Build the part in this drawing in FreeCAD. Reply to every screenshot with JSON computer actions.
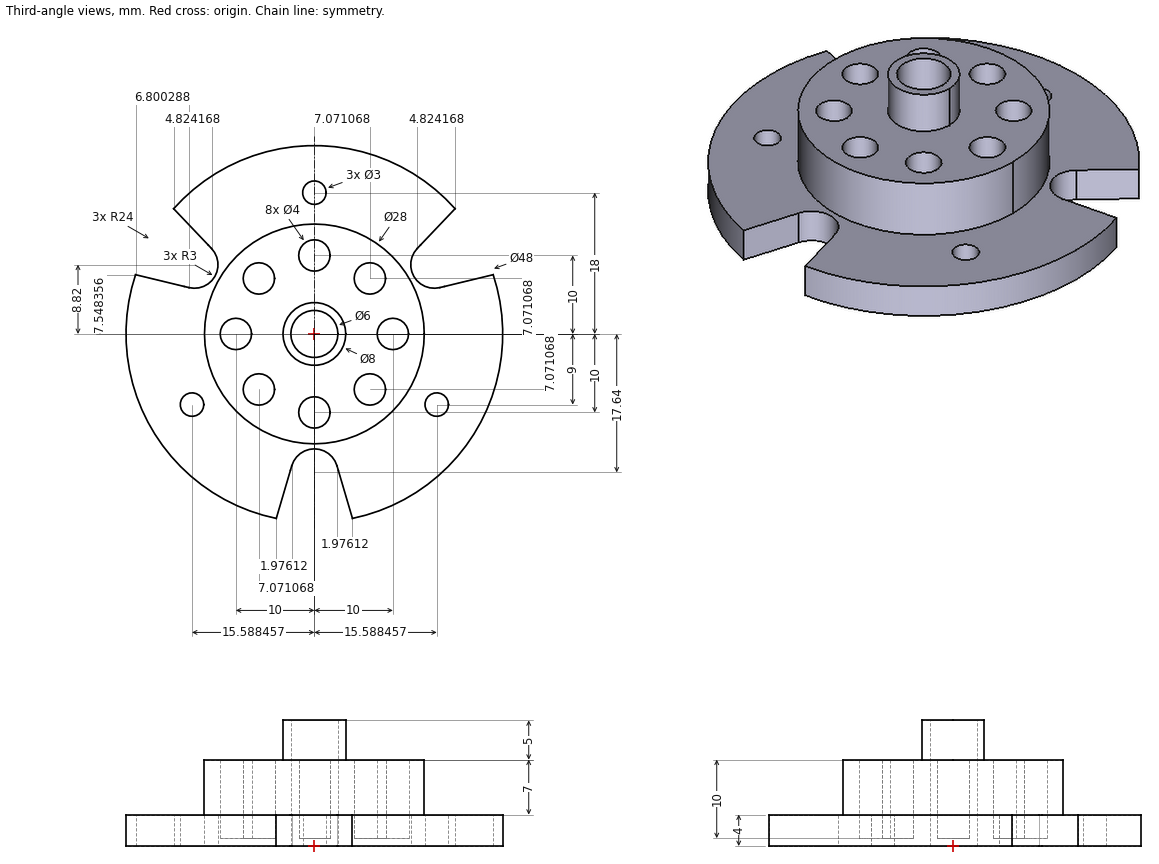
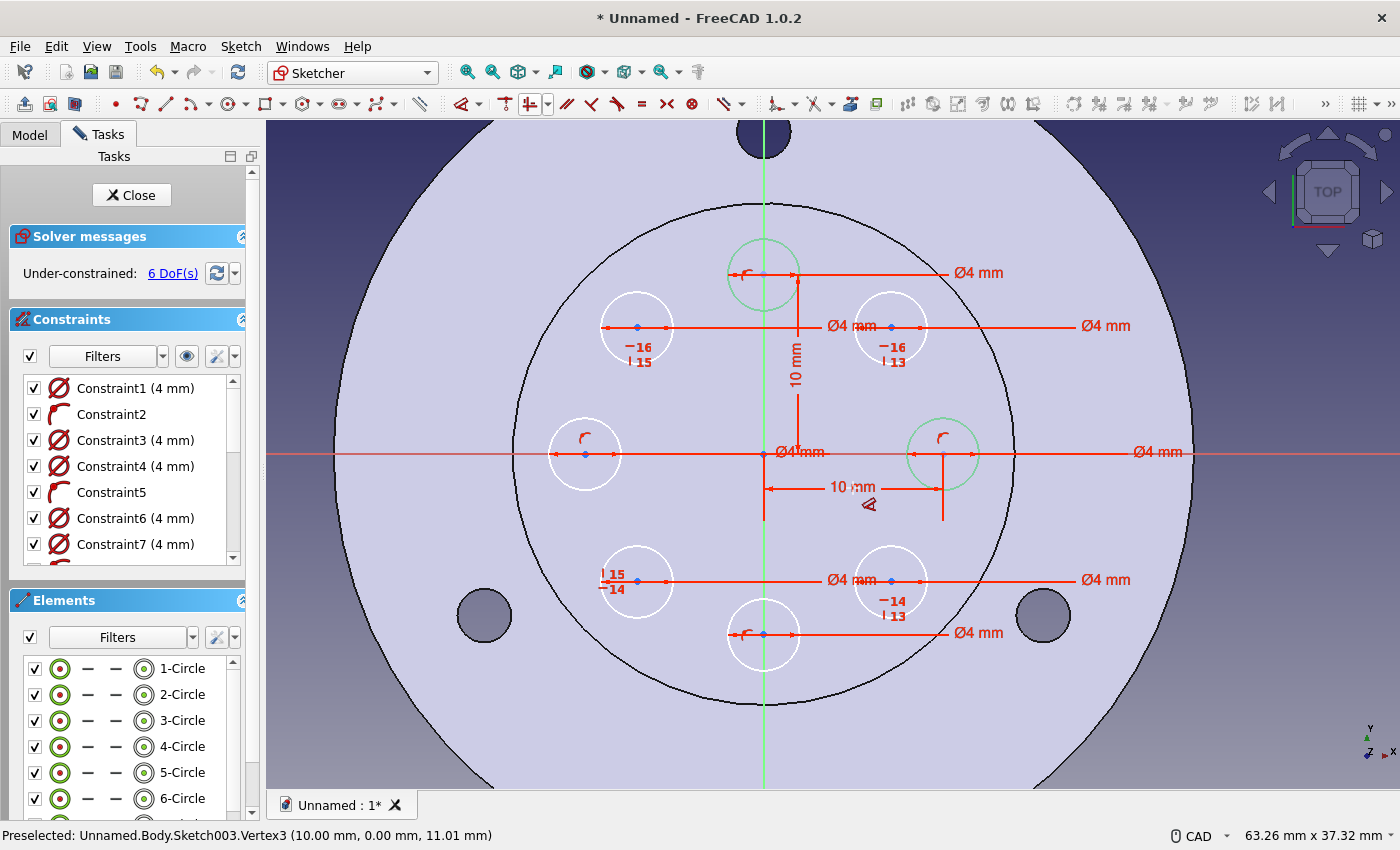
{"action": "left_click", "coordinate": [764, 635]}
{"action": "left_click", "coordinate": [798, 545]}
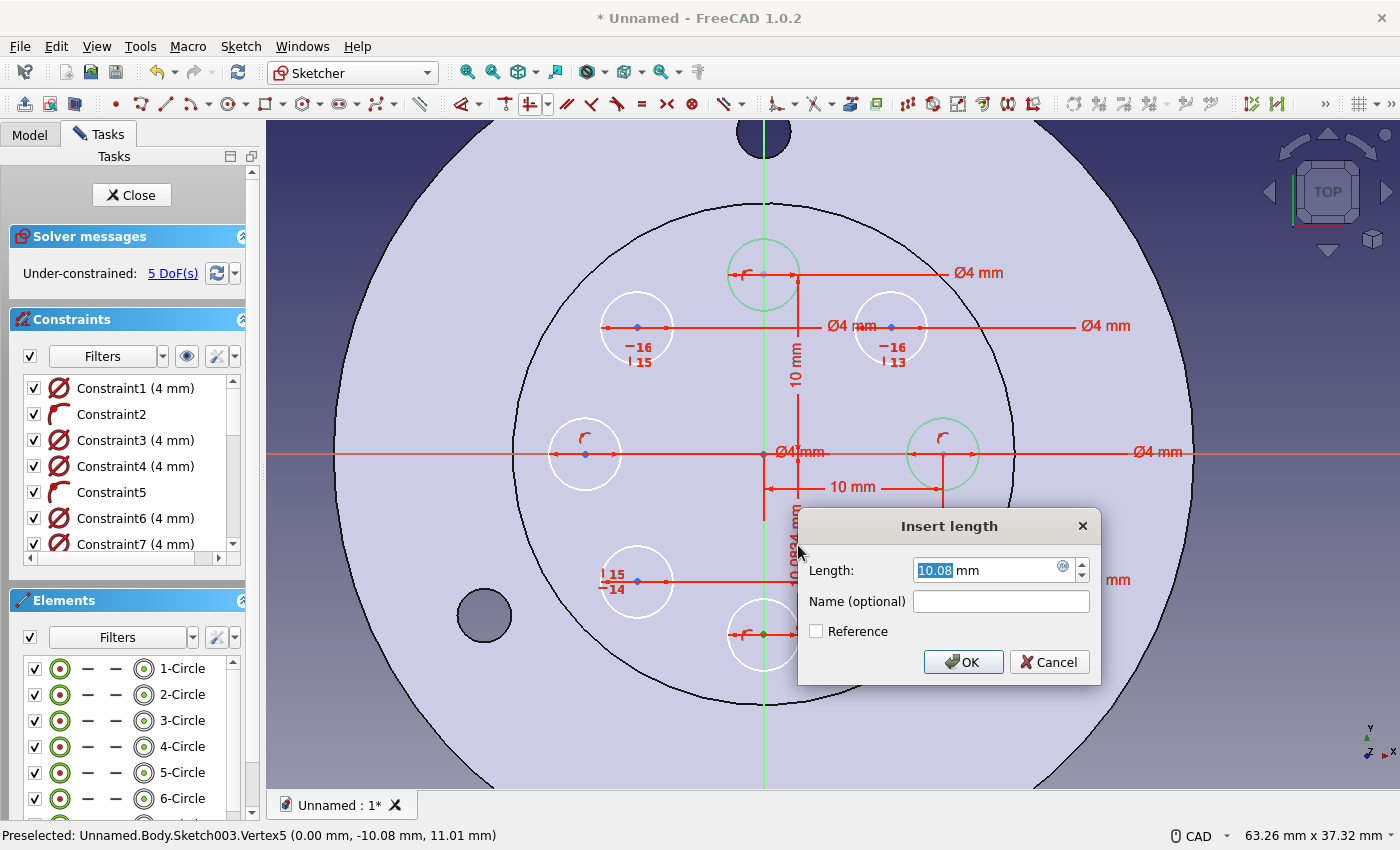
{"action": "type", "text": "10"}
{"action": "key", "text": "Return"}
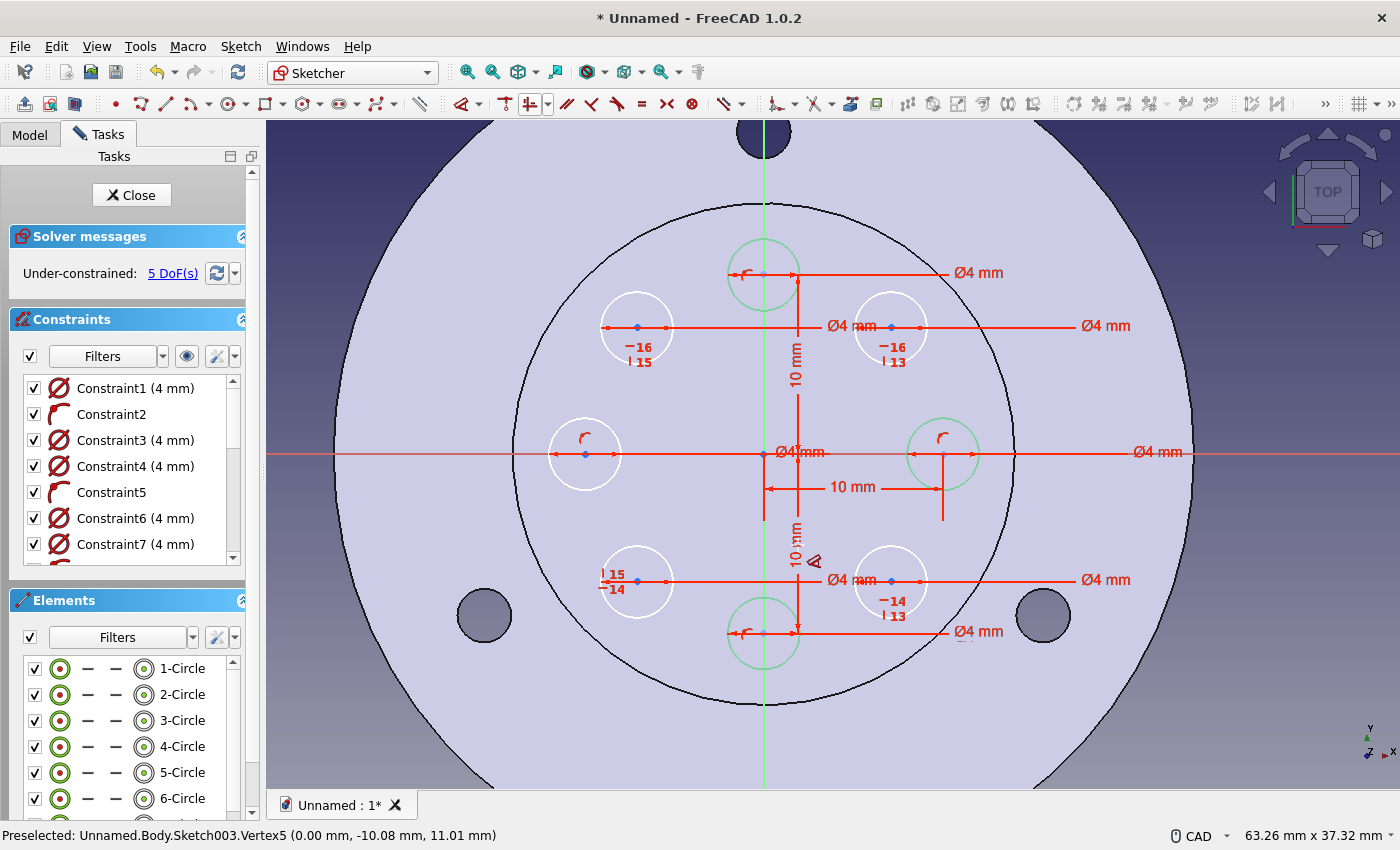
{"action": "left_click", "coordinate": [585, 454]}
{"action": "left_click", "coordinate": [674, 488]}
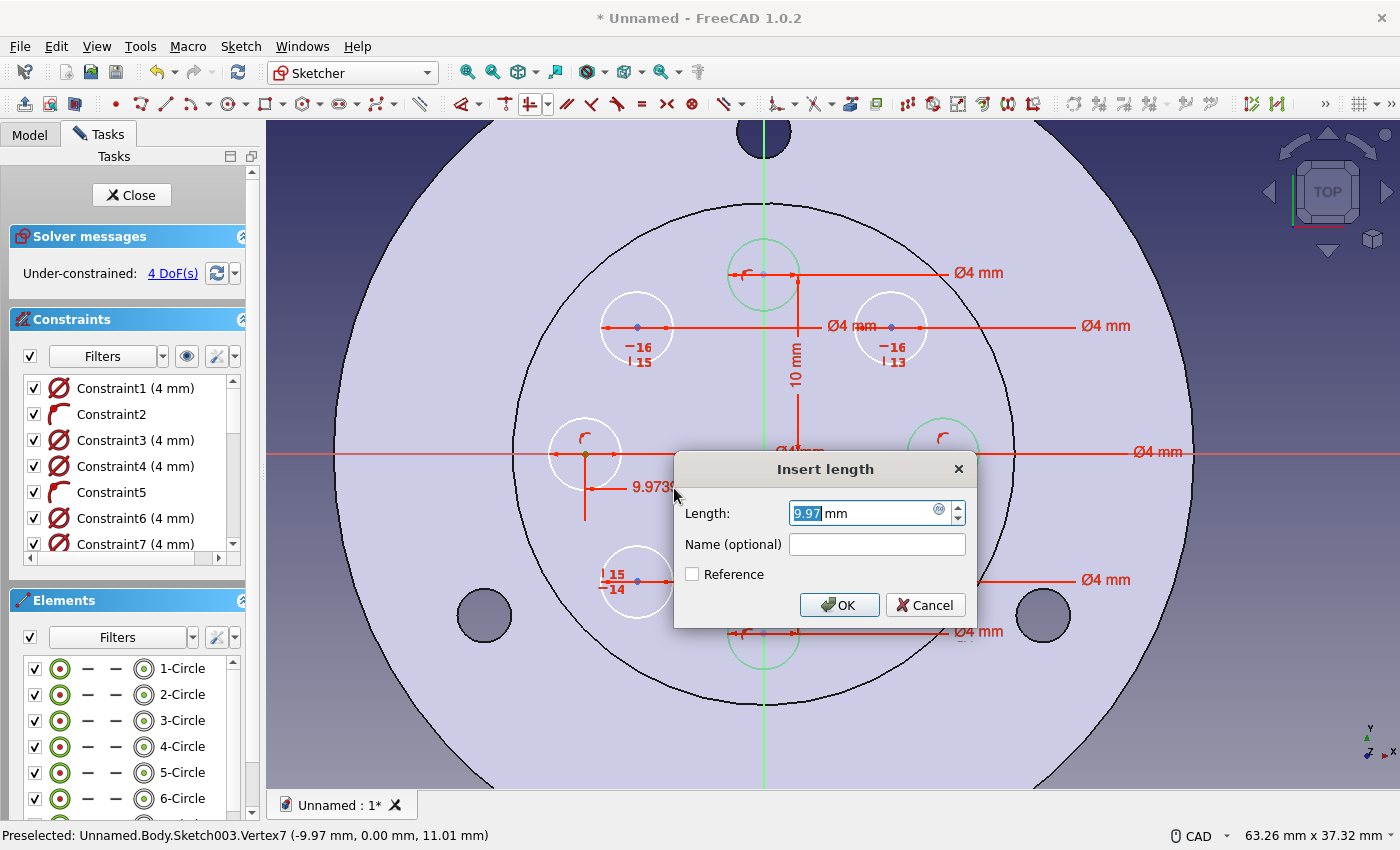
{"action": "type", "text": "10"}
{"action": "key", "text": "Return"}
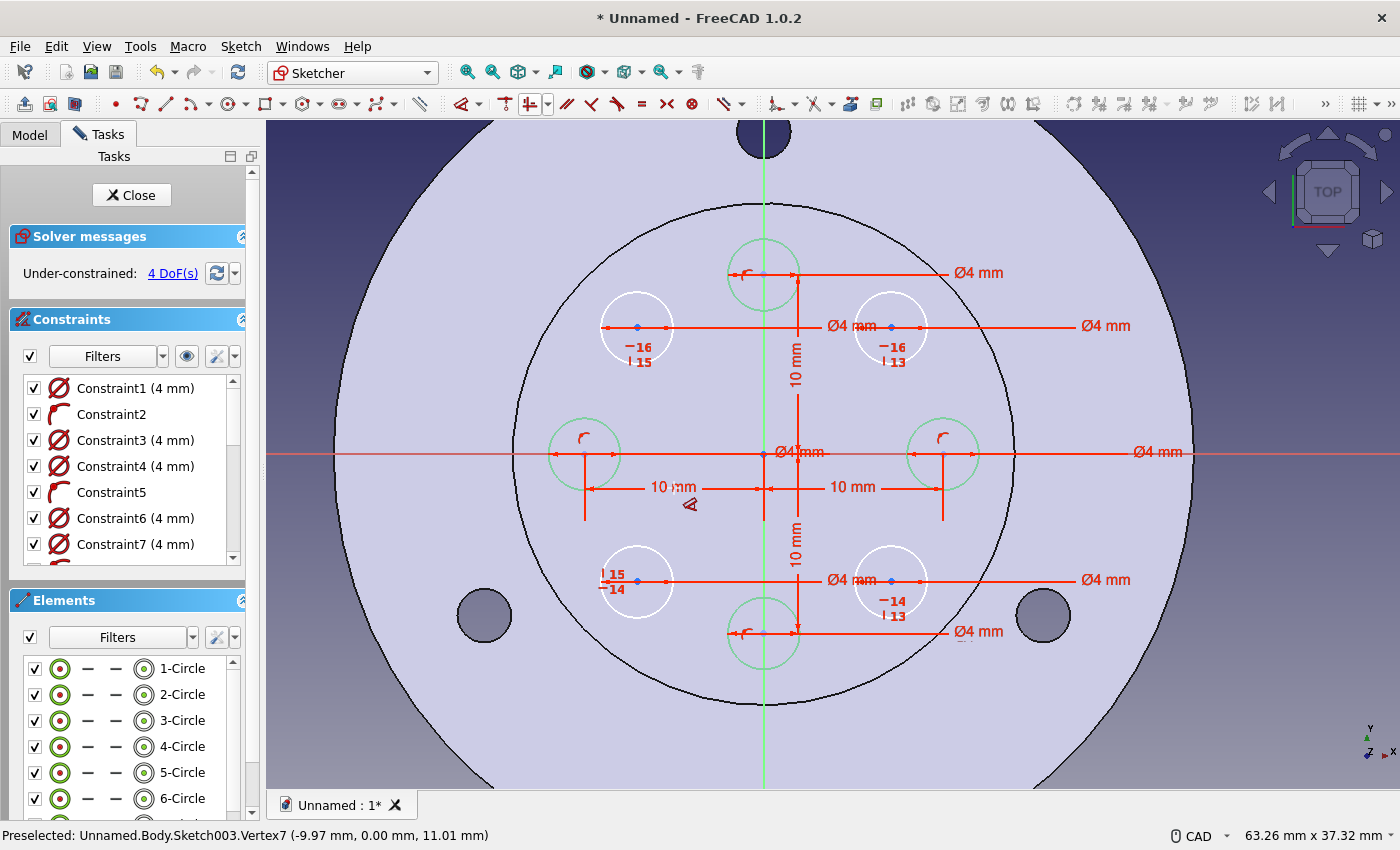
{"action": "left_click", "coordinate": [891, 328]}
{"action": "left_click", "coordinate": [827, 294]}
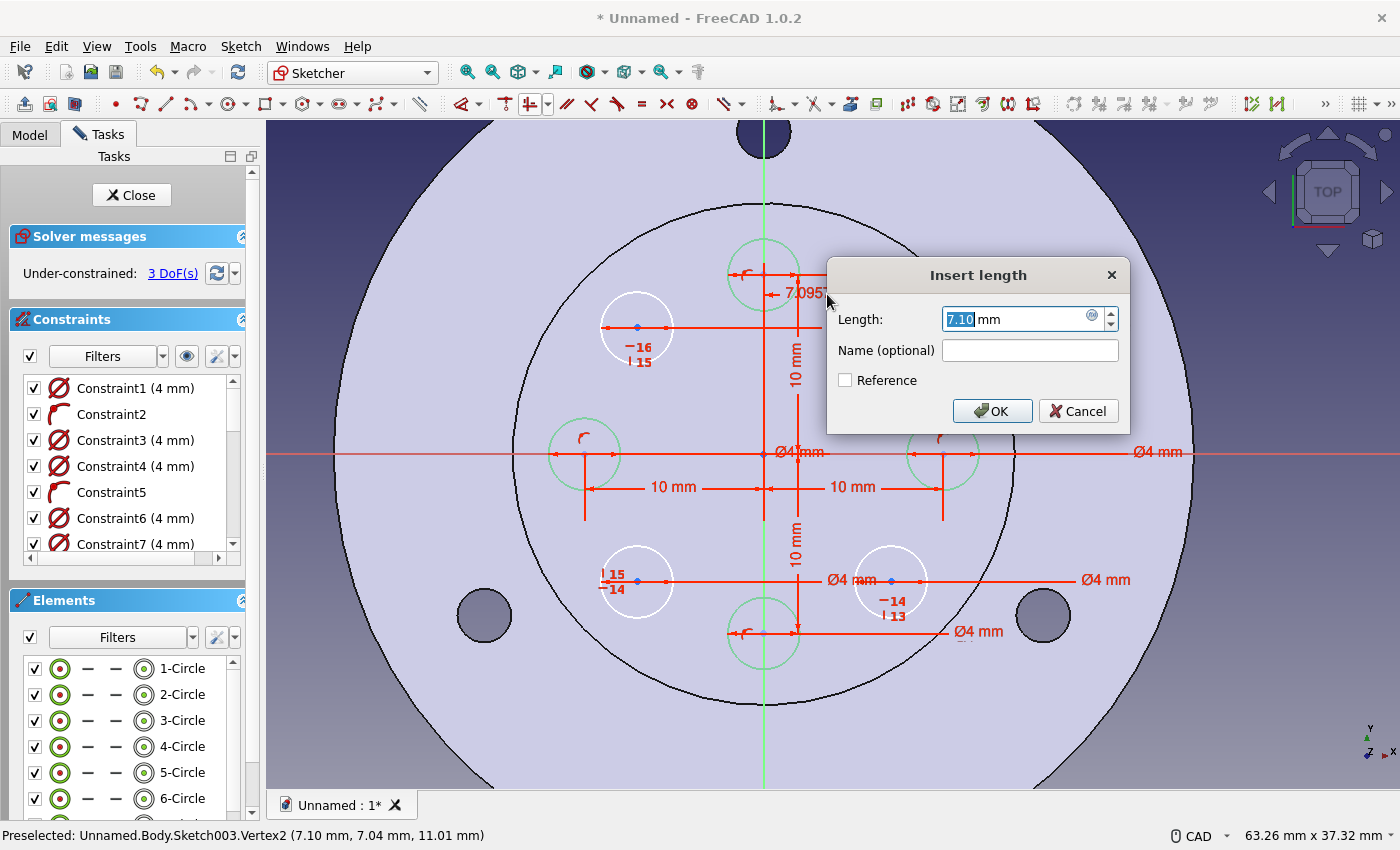
{"action": "type", "text": "7.071068"}
{"action": "key", "text": "Return"}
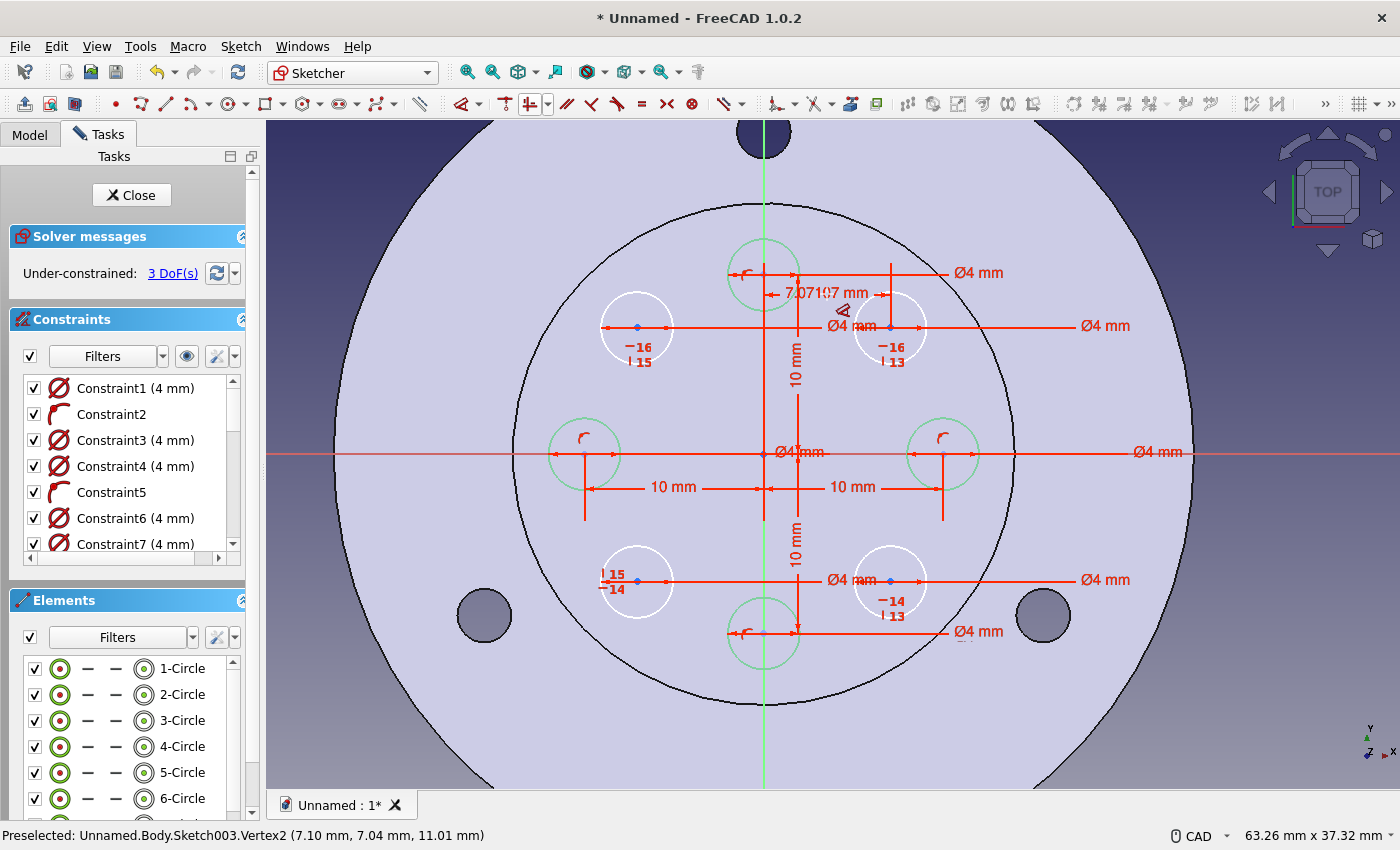
{"action": "left_click", "coordinate": [891, 328]}
{"action": "left_click", "coordinate": [925, 391]}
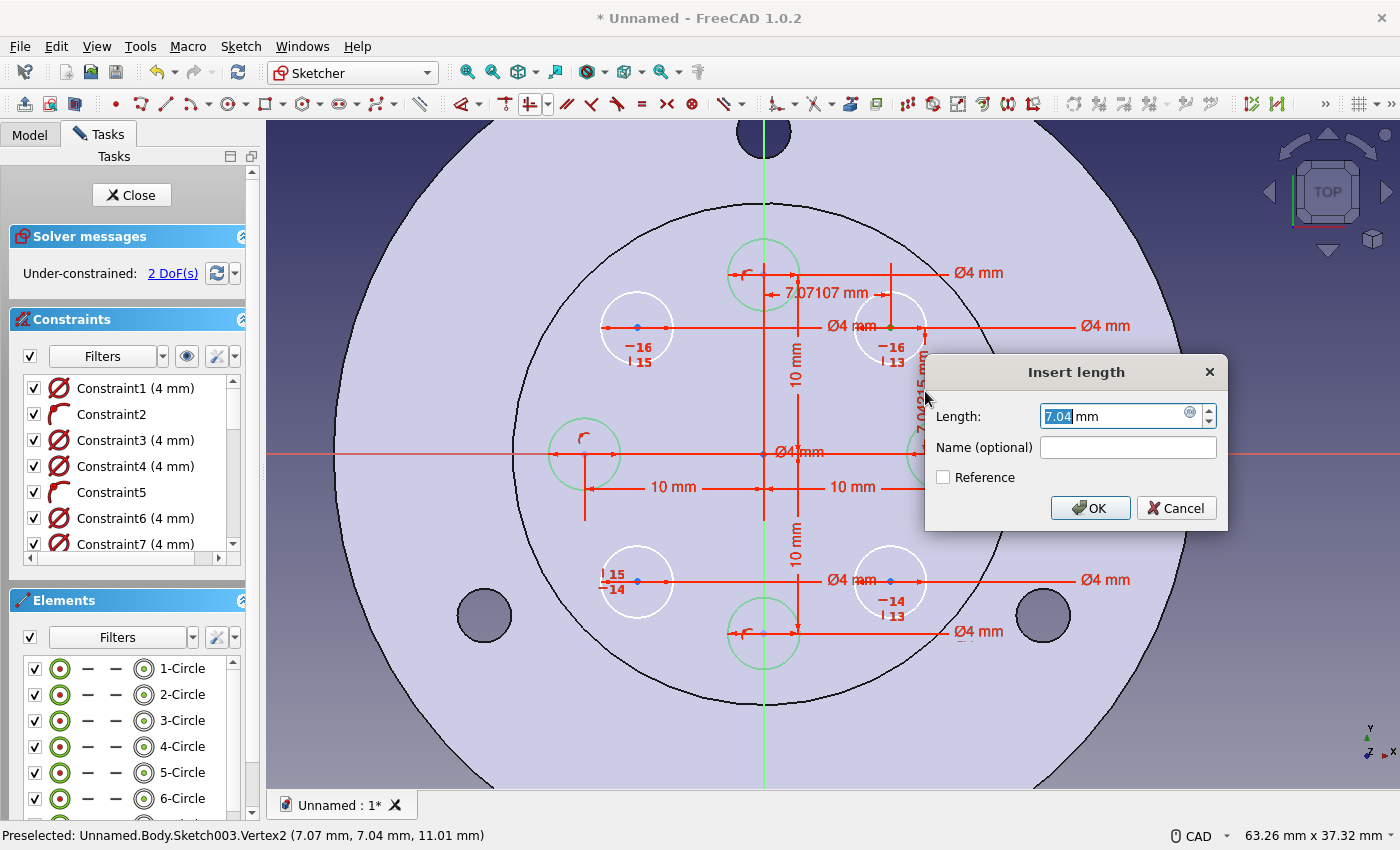
{"action": "type", "text": "7.071068"}
{"action": "key", "text": "Return"}